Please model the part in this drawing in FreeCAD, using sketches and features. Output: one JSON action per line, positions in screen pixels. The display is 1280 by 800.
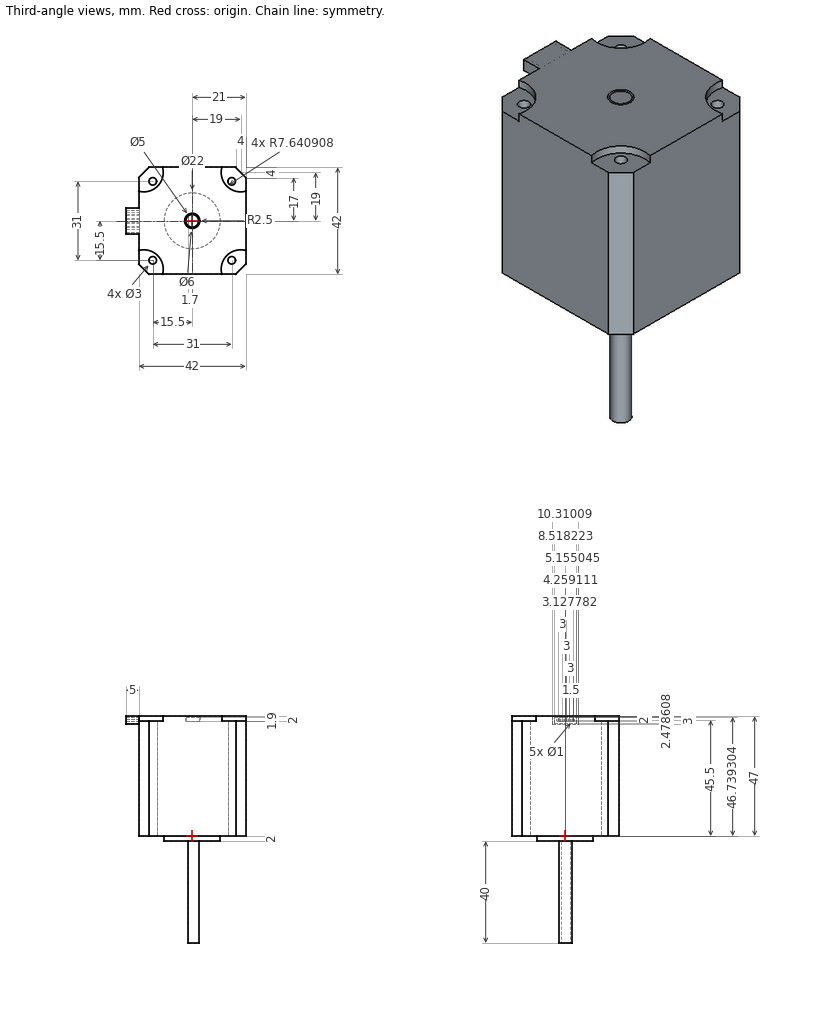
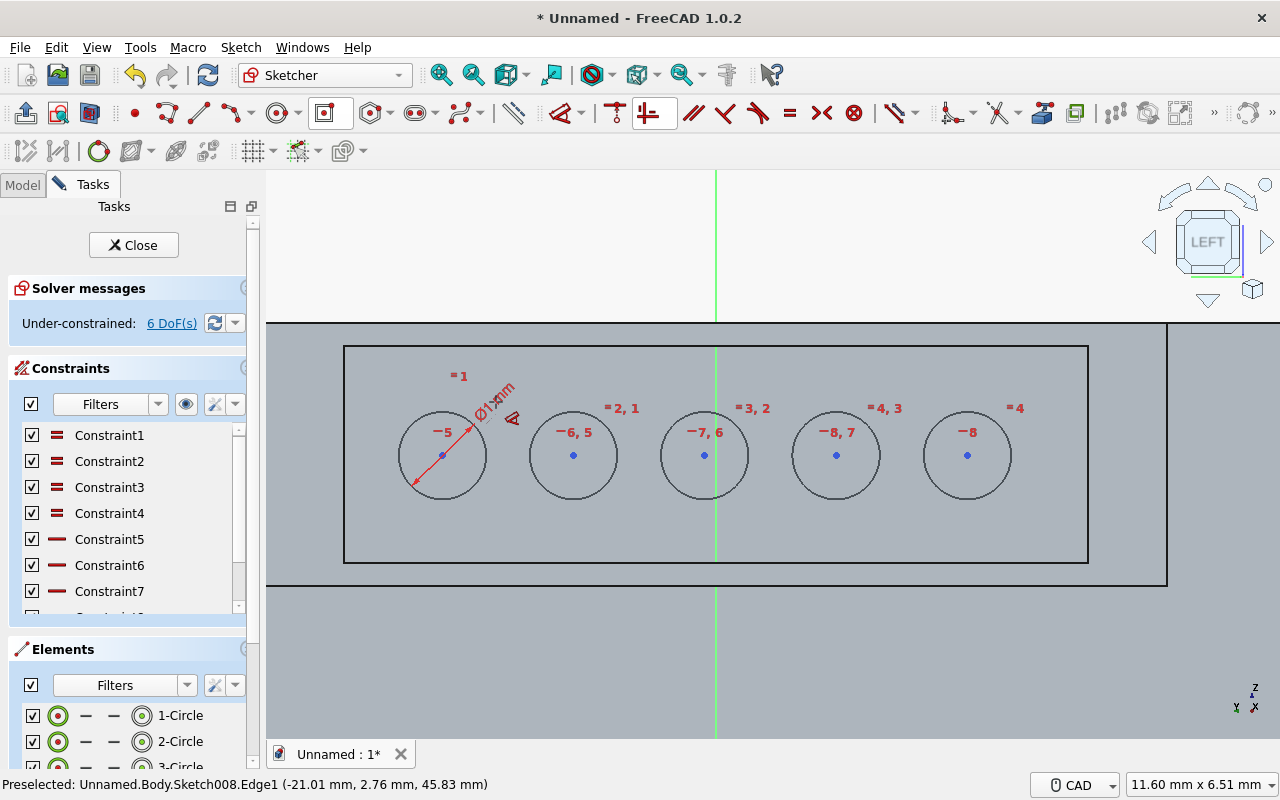
{"action": "left_click", "coordinate": [443, 456]}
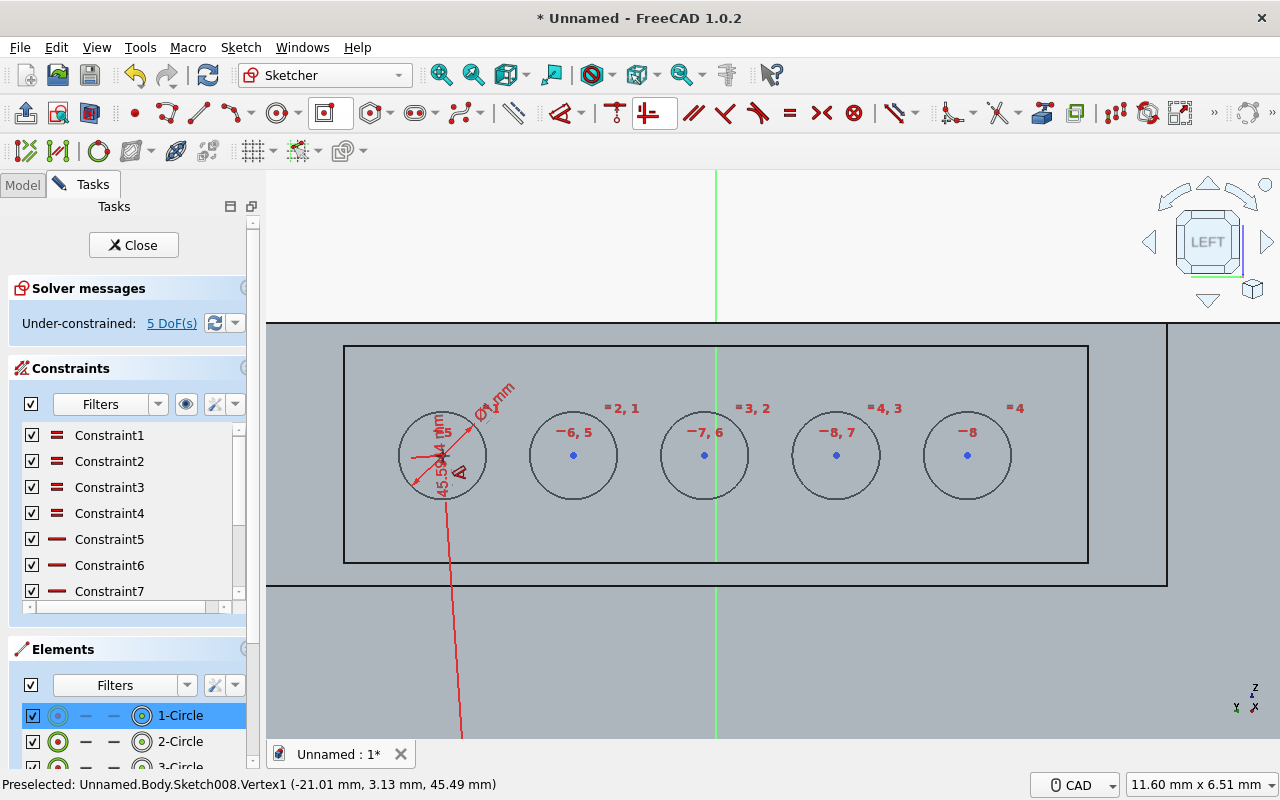
{"action": "left_click", "coordinate": [705, 456]}
{"action": "left_click", "coordinate": [513, 490]}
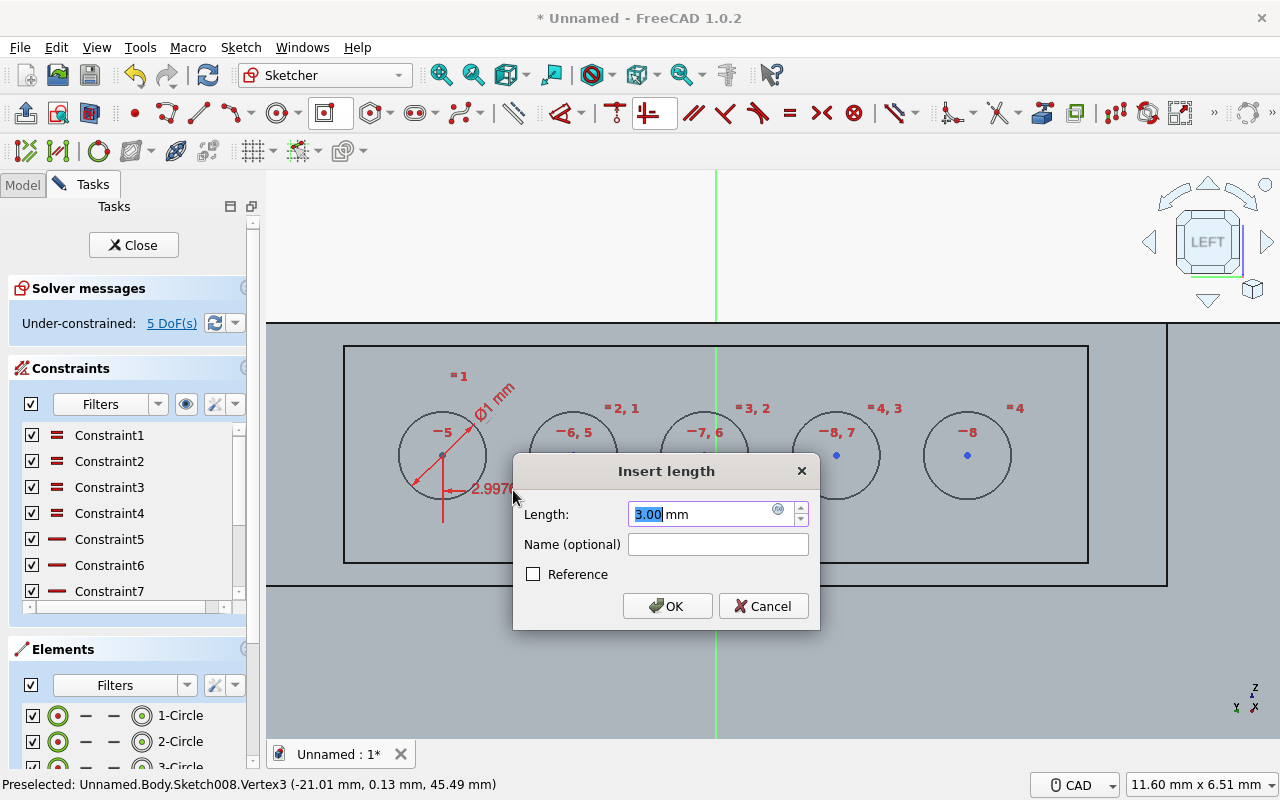
{"action": "type", "text": "3"}
{"action": "key", "text": "Return"}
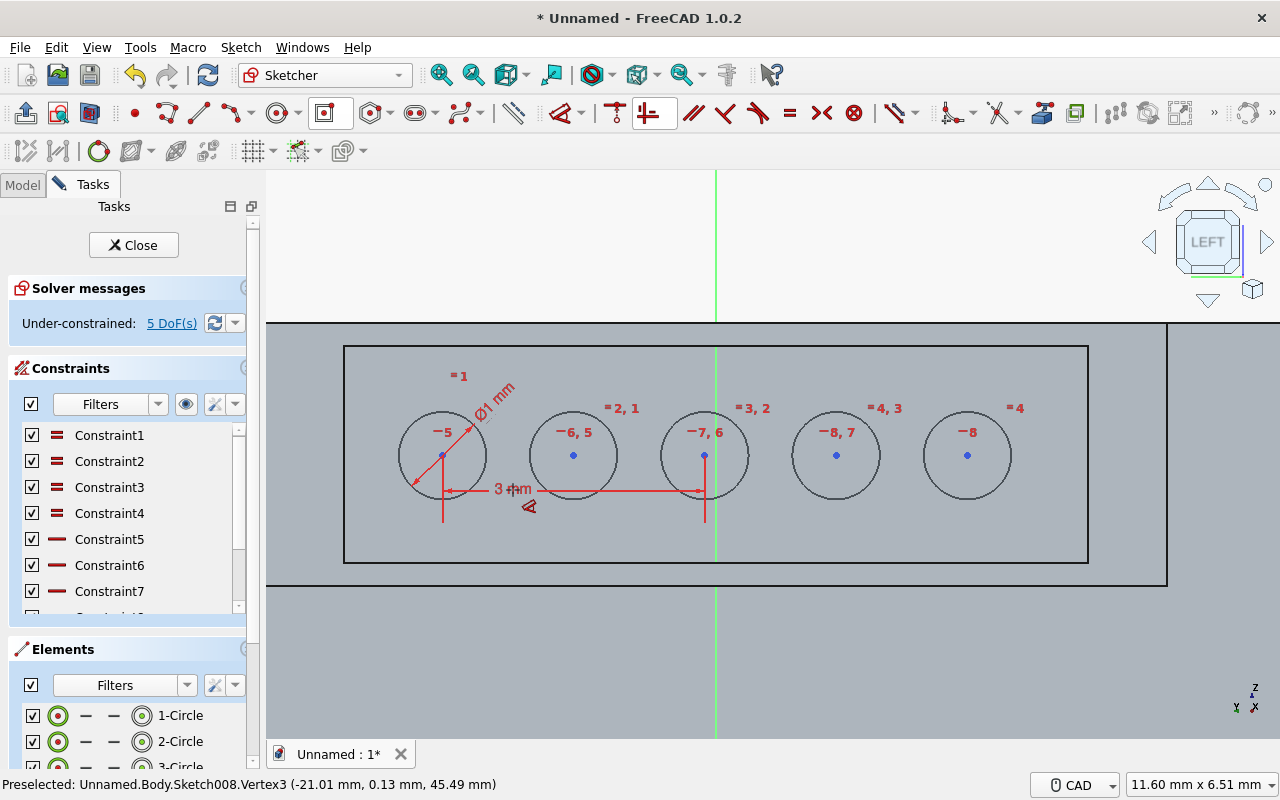
{"action": "left_click", "coordinate": [574, 456]}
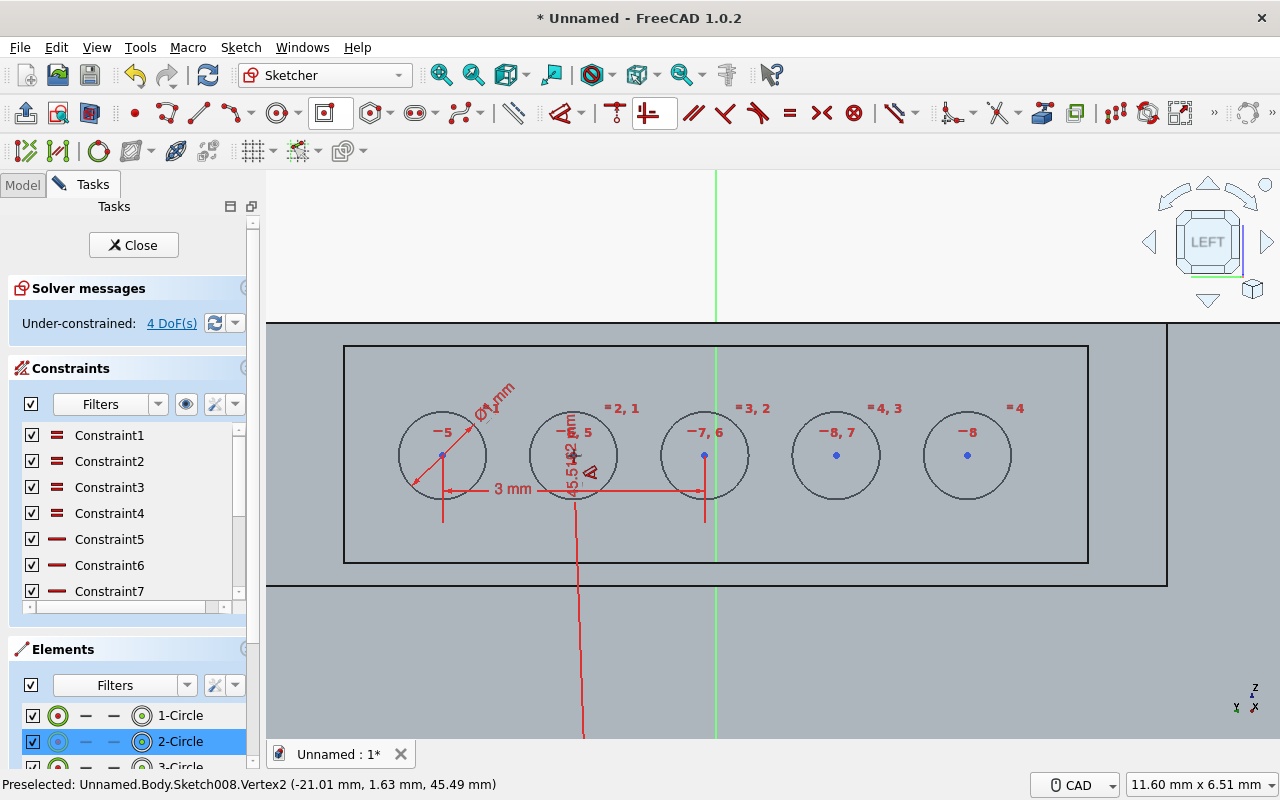
{"action": "left_click", "coordinate": [836, 456]}
{"action": "left_click", "coordinate": [644, 490]}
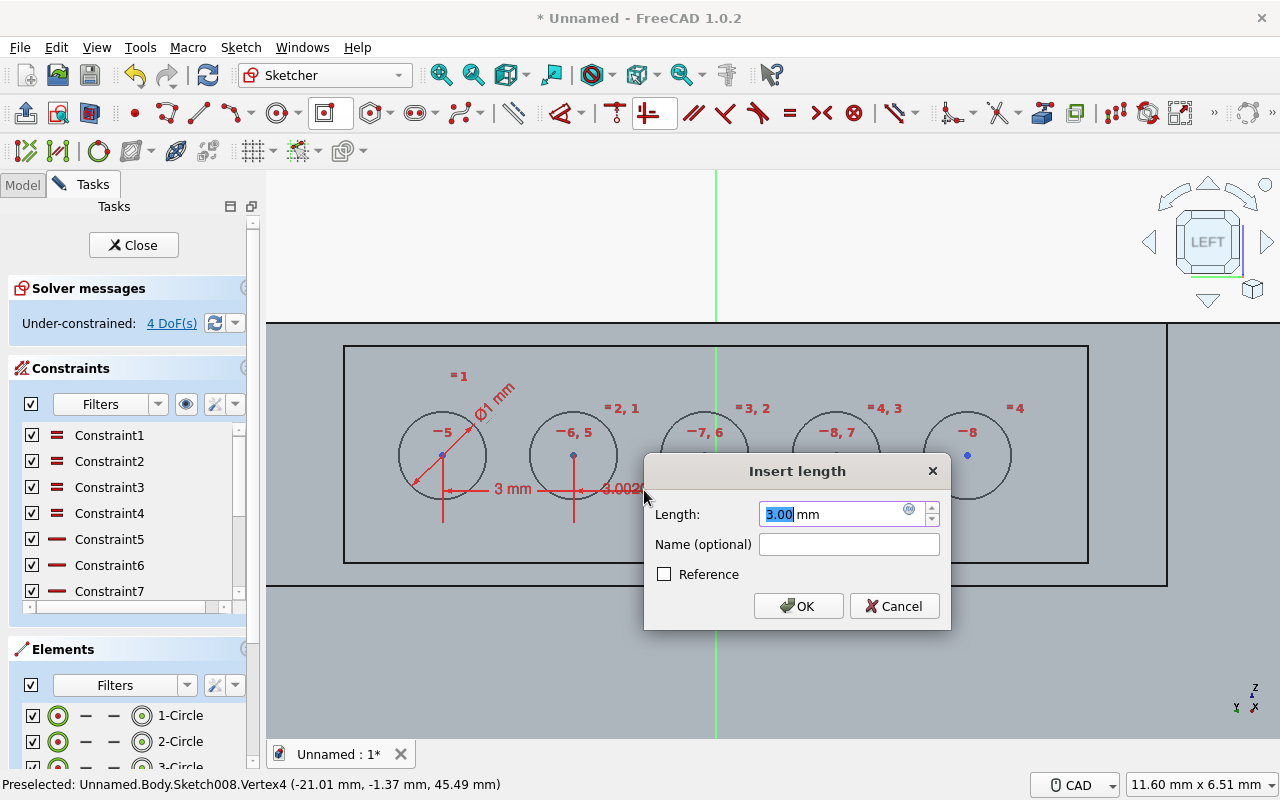
{"action": "type", "text": "3"}
{"action": "key", "text": "Return"}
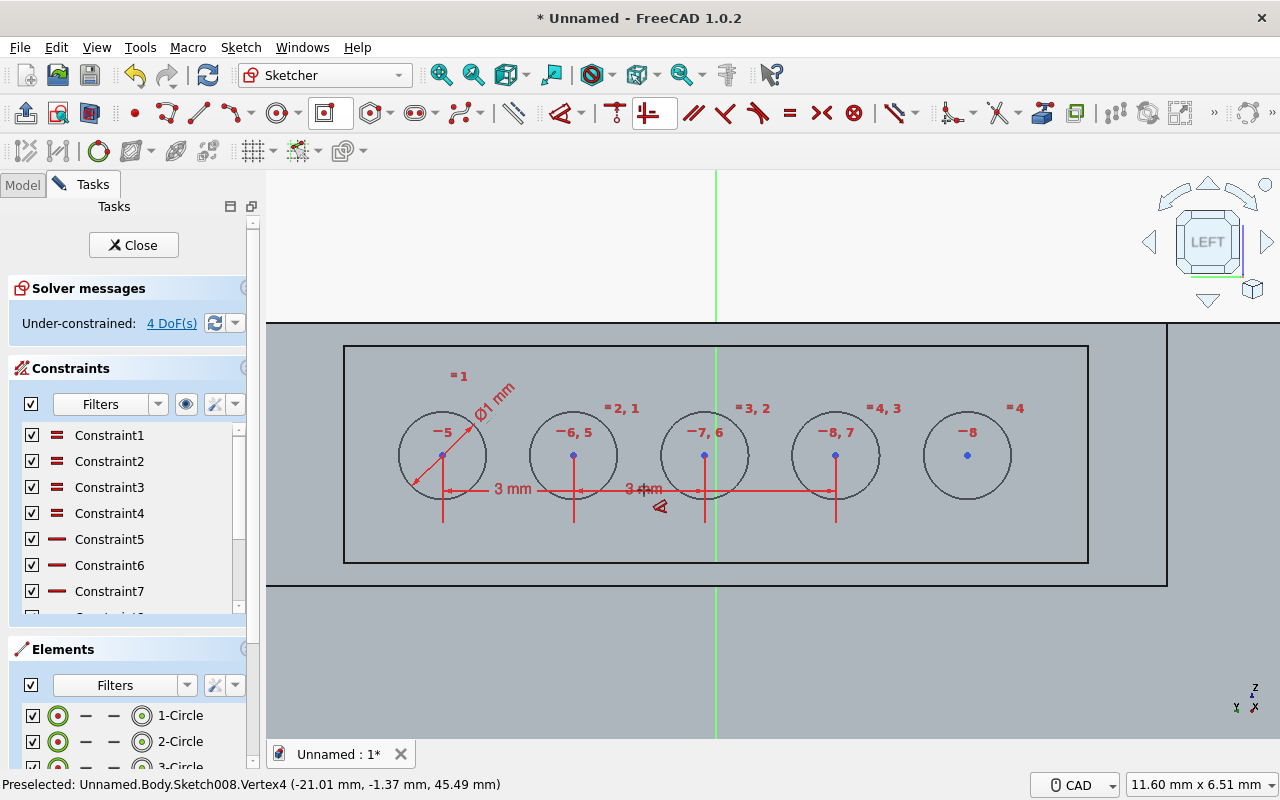
{"action": "left_click", "coordinate": [705, 456]}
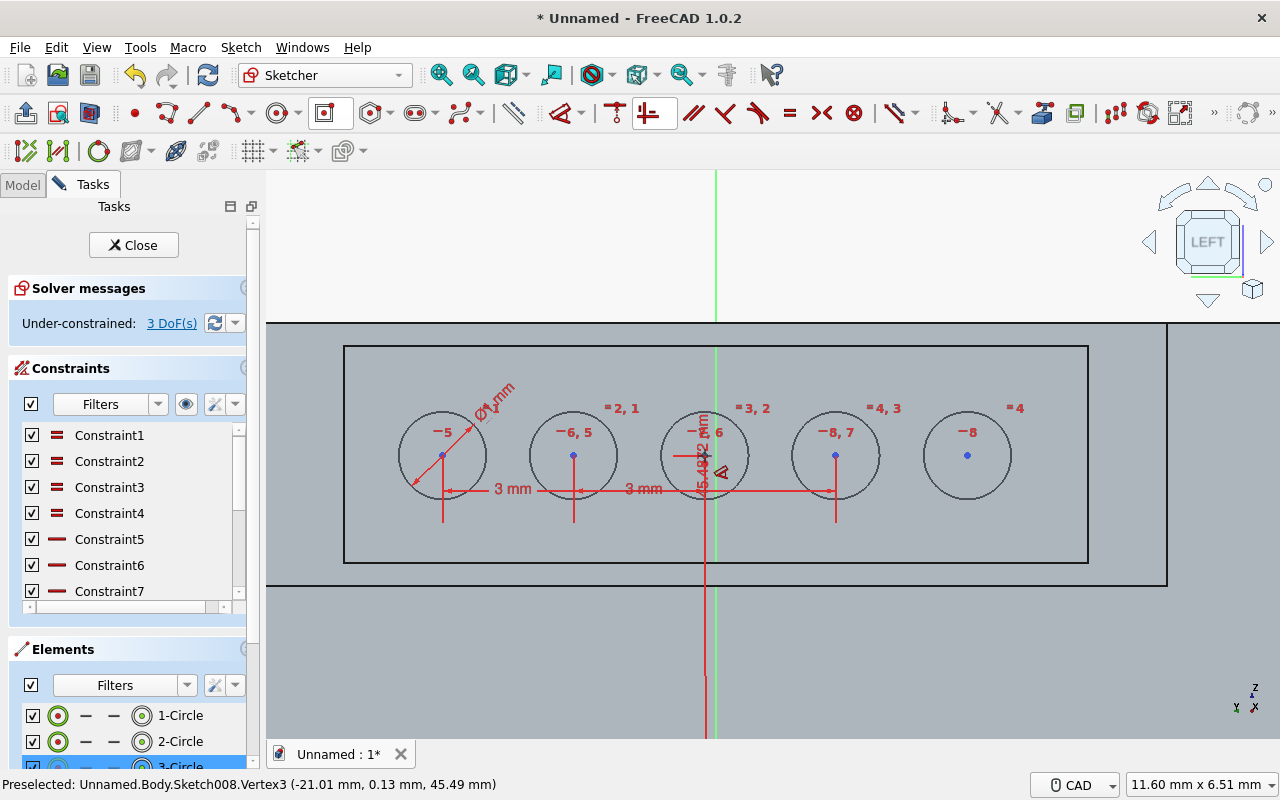
{"action": "left_click", "coordinate": [967, 456]}
{"action": "left_click", "coordinate": [776, 490]}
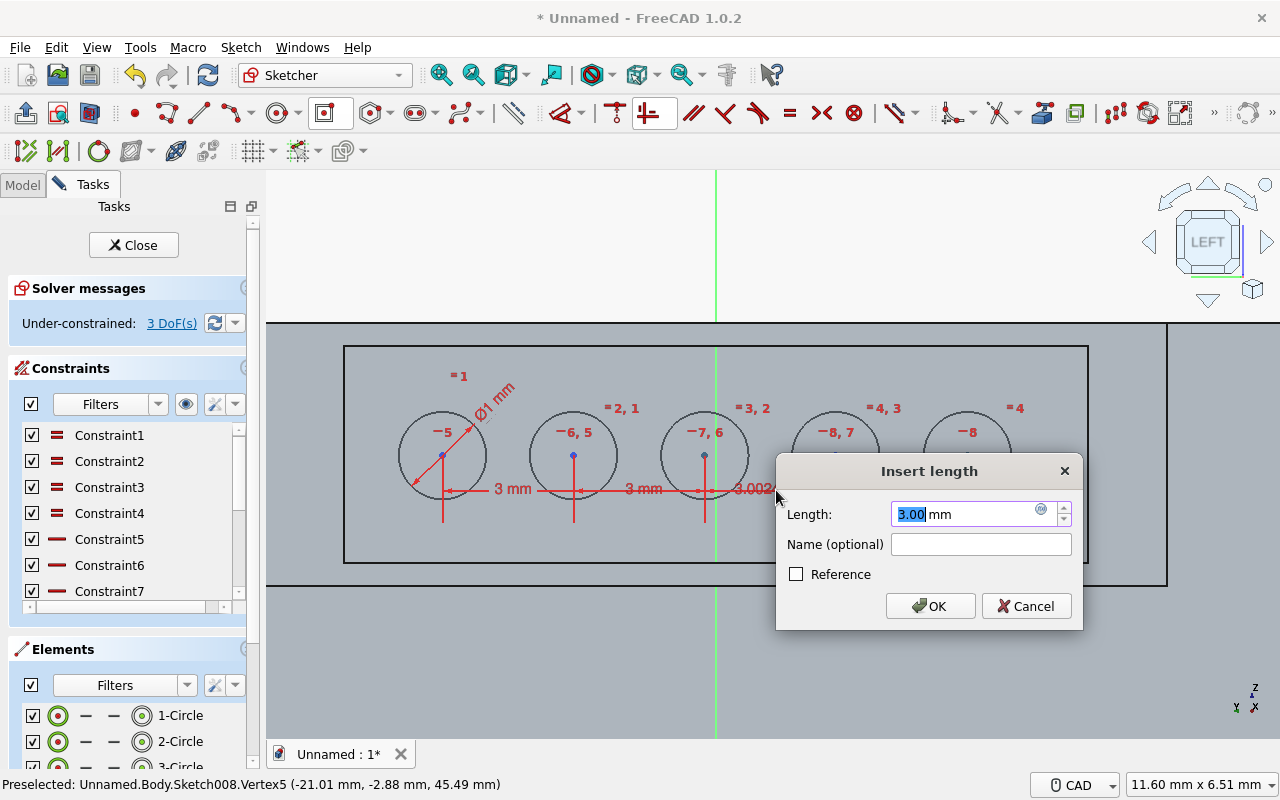
{"action": "type", "text": "3"}
{"action": "key", "text": "Return"}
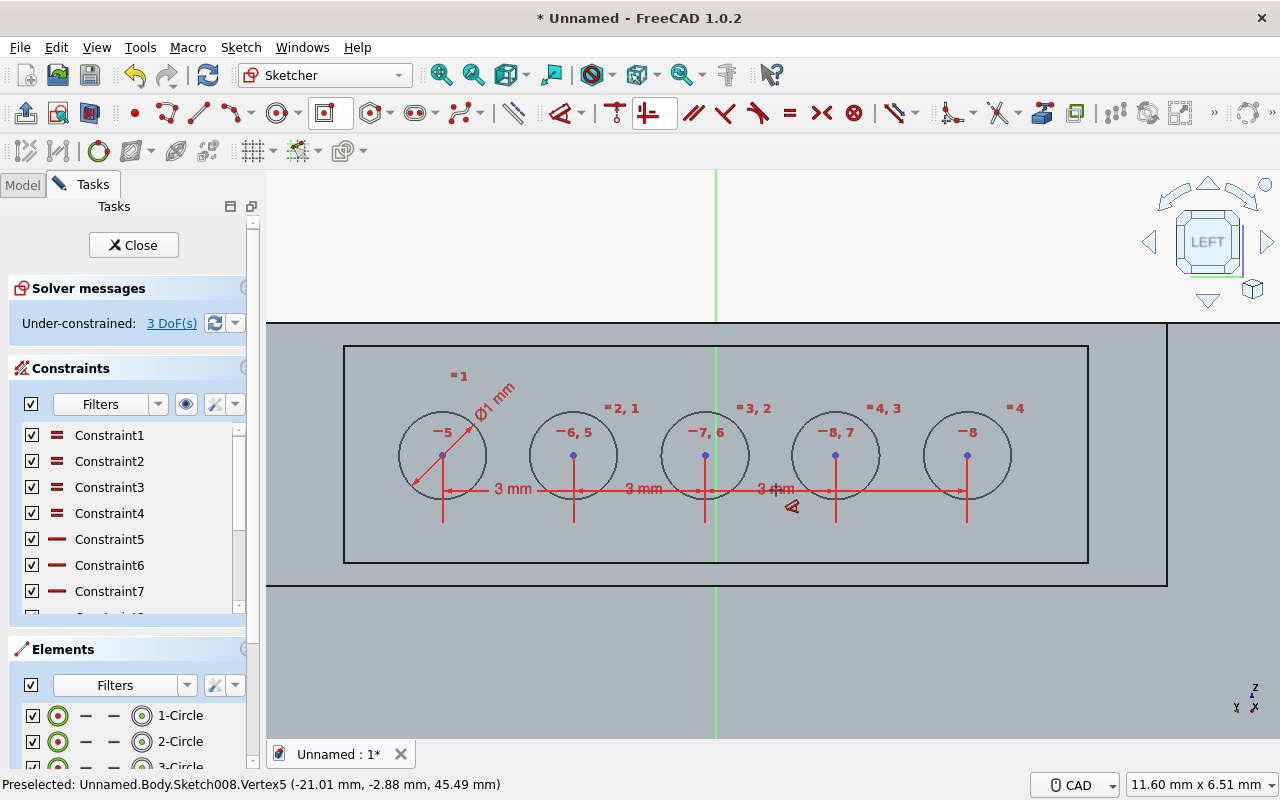
{"action": "left_click", "coordinate": [443, 456]}
{"action": "left_click", "coordinate": [409, 583]}